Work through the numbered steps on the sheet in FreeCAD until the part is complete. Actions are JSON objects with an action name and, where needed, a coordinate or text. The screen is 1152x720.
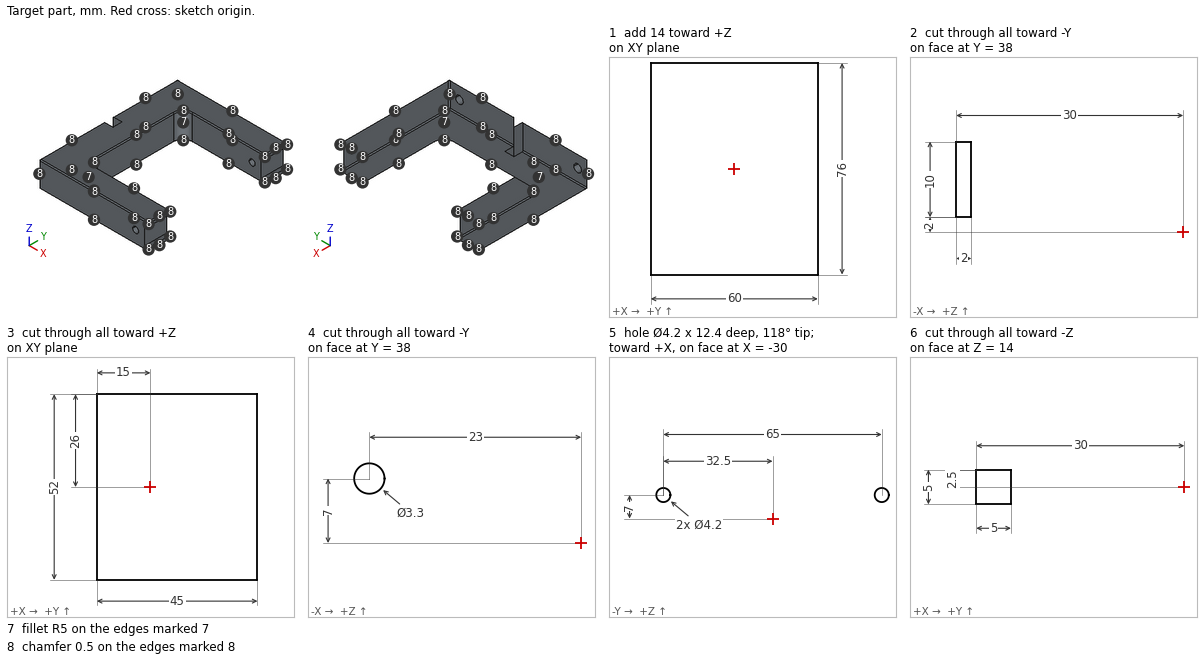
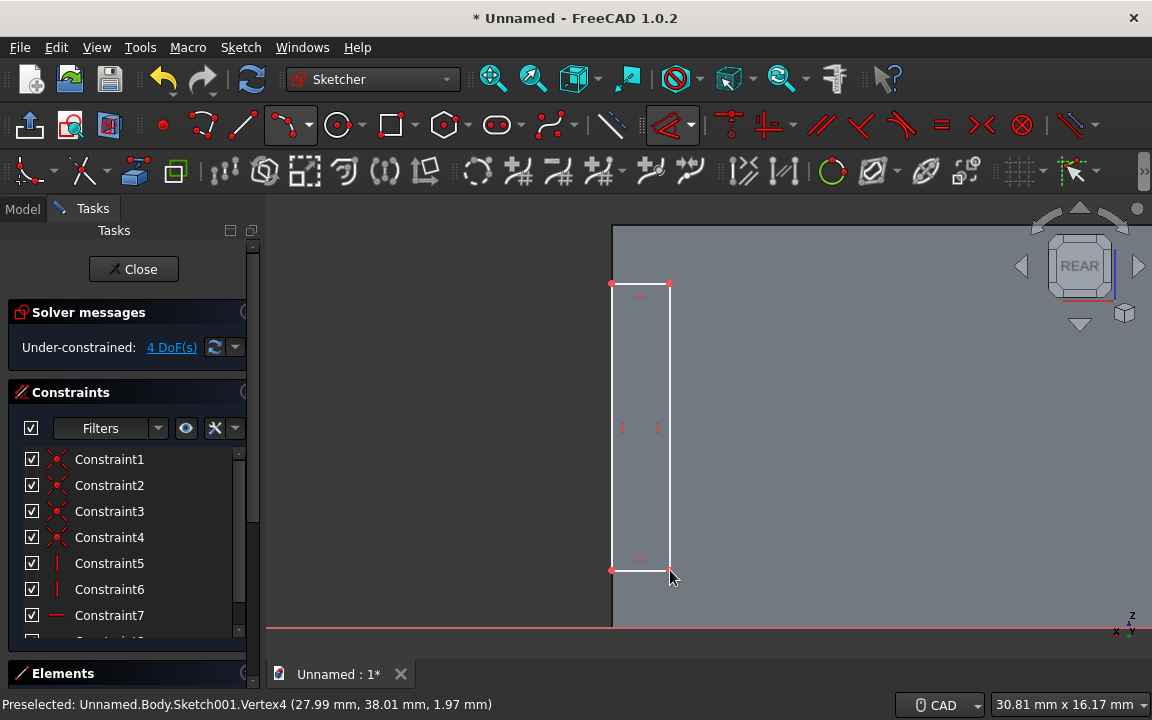
{"action": "left_click", "coordinate": [629, 571]}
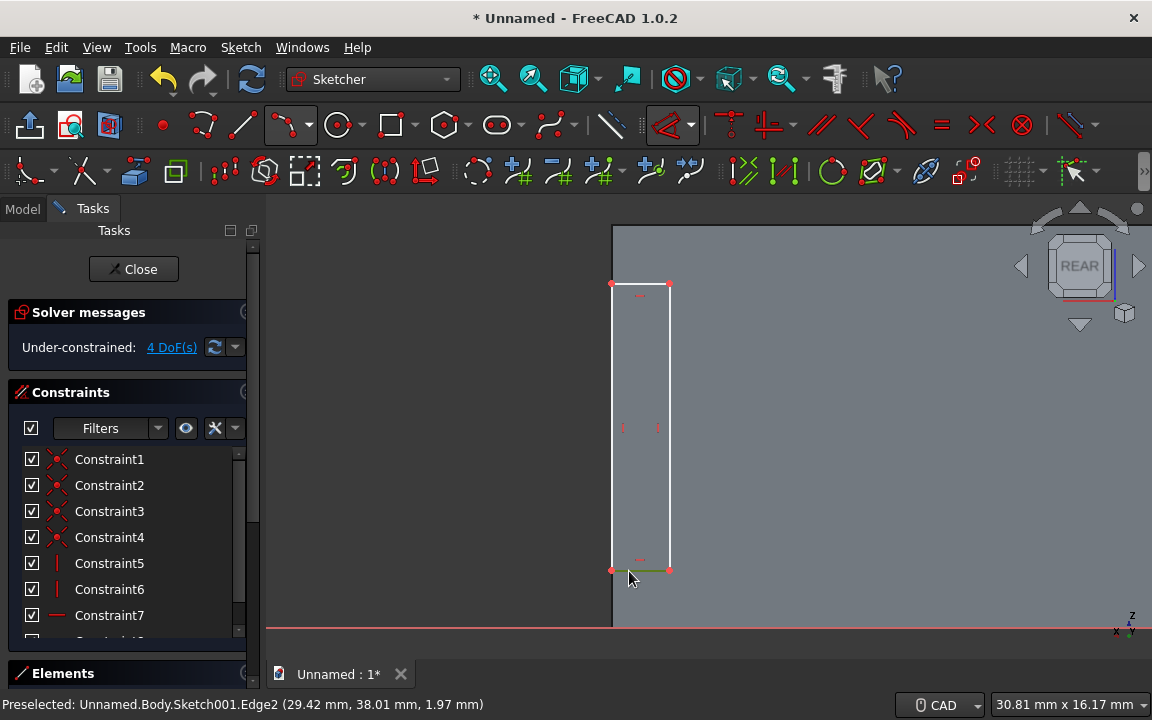
{"action": "key", "text": "l"}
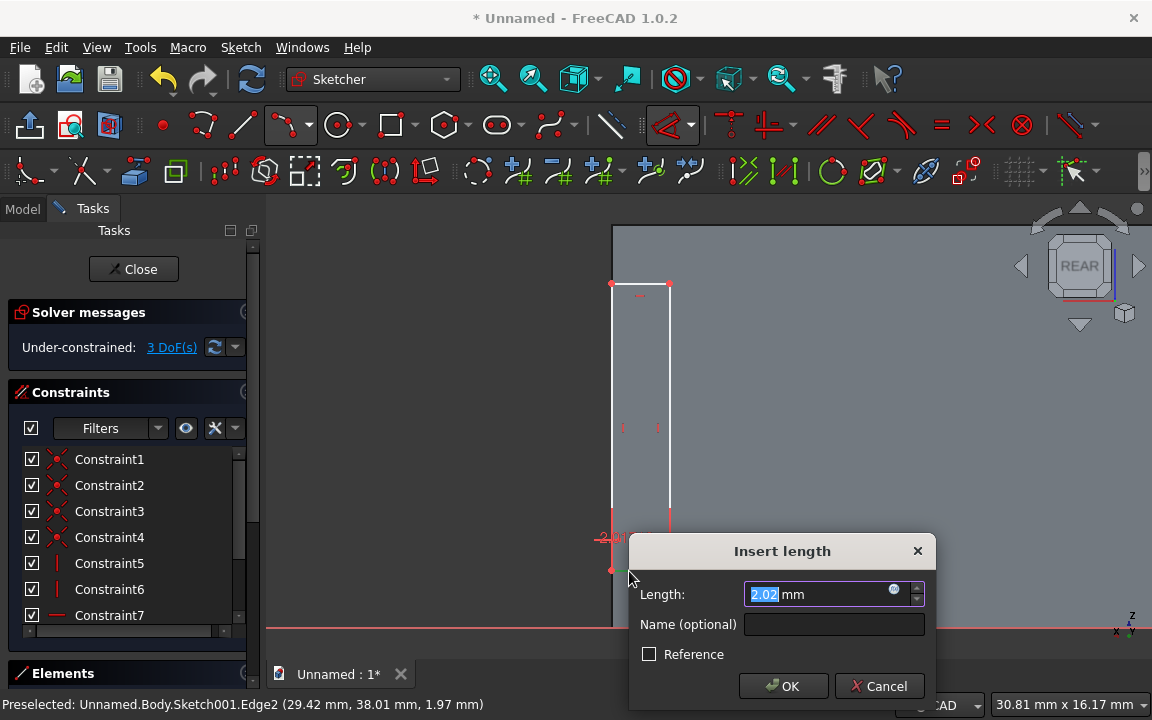
{"action": "type", "text": "2"}
{"action": "key", "text": "Return"}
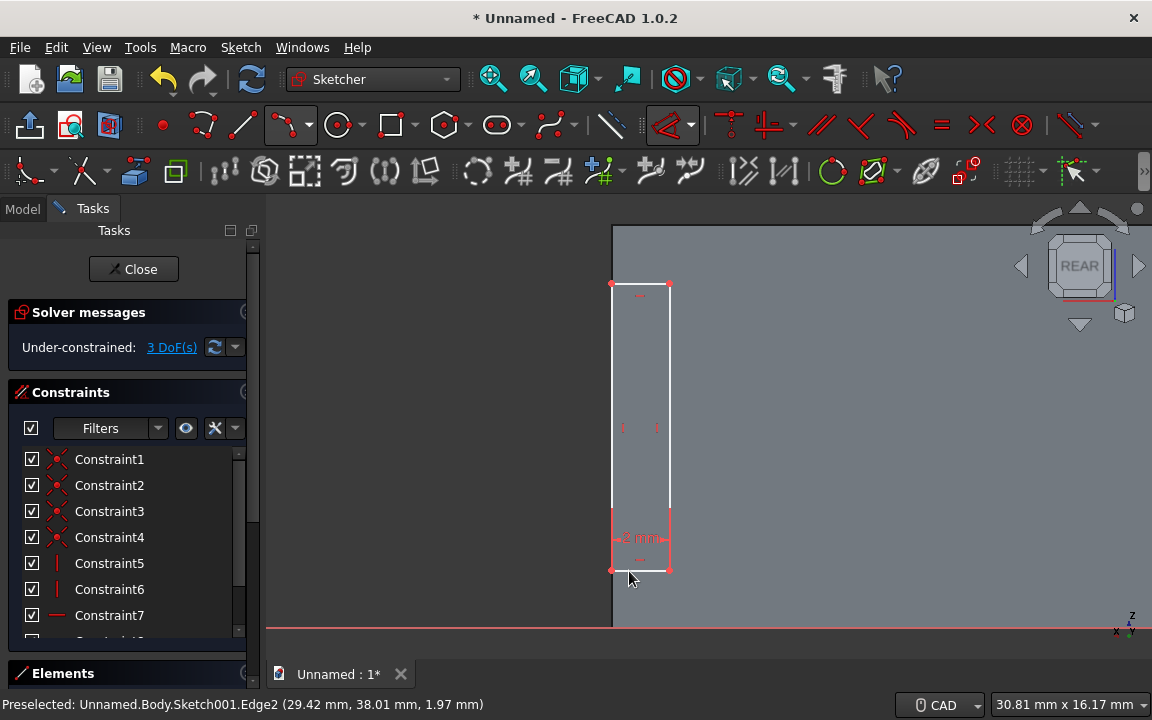
{"action": "left_click", "coordinate": [612, 370]}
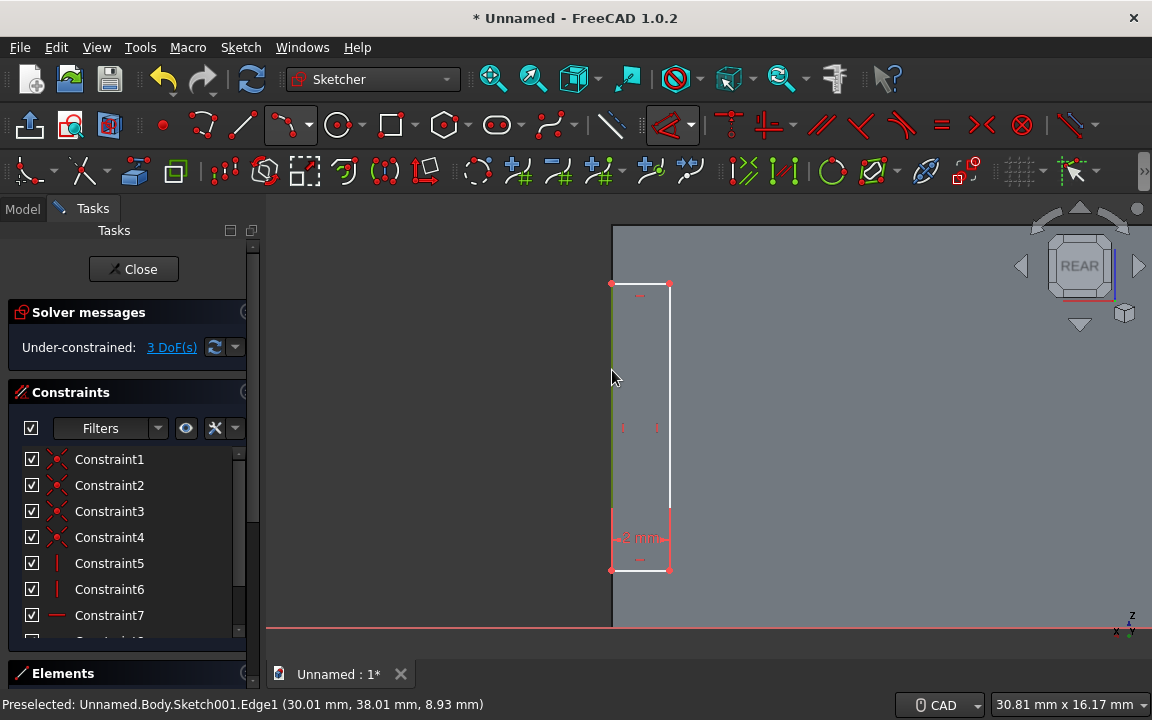
{"action": "key", "text": "i"}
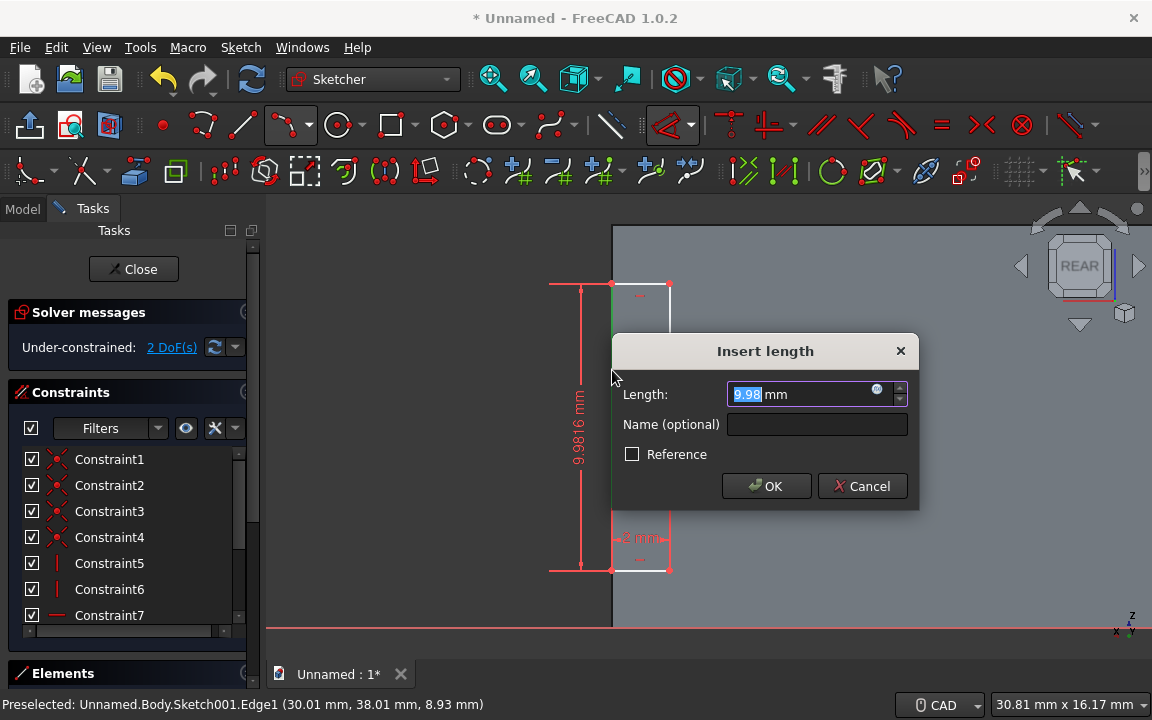
{"action": "type", "text": "10"}
{"action": "key", "text": "Return"}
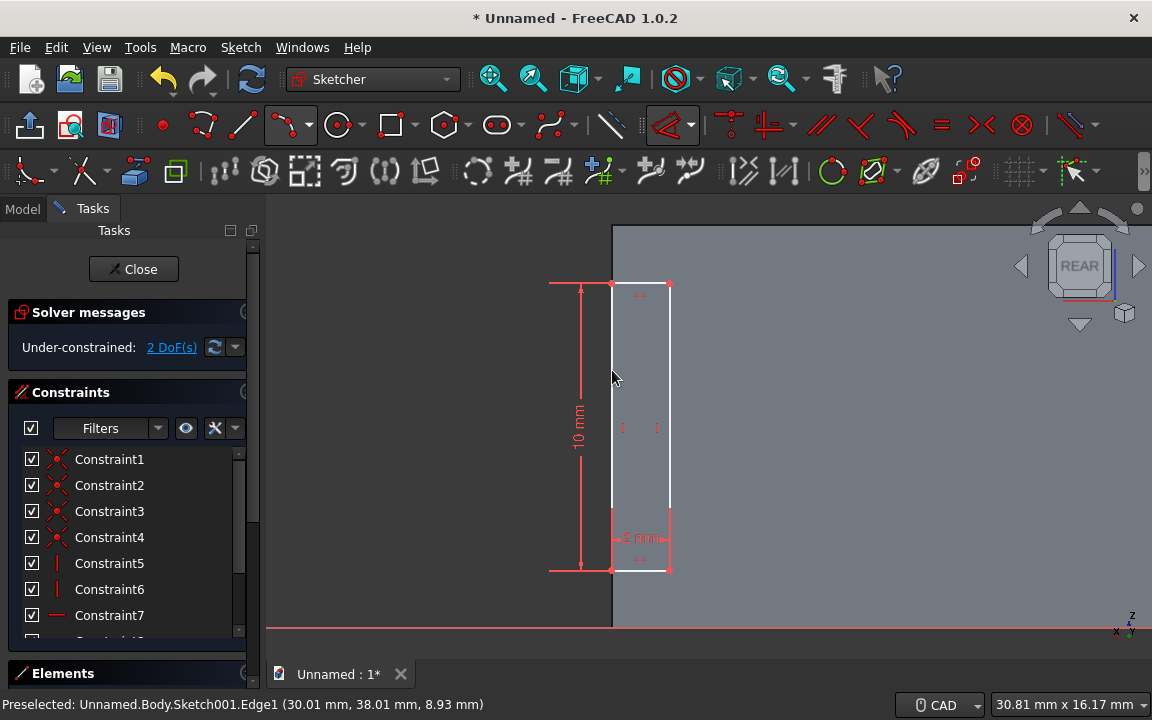
{"action": "left_click", "coordinate": [612, 571]}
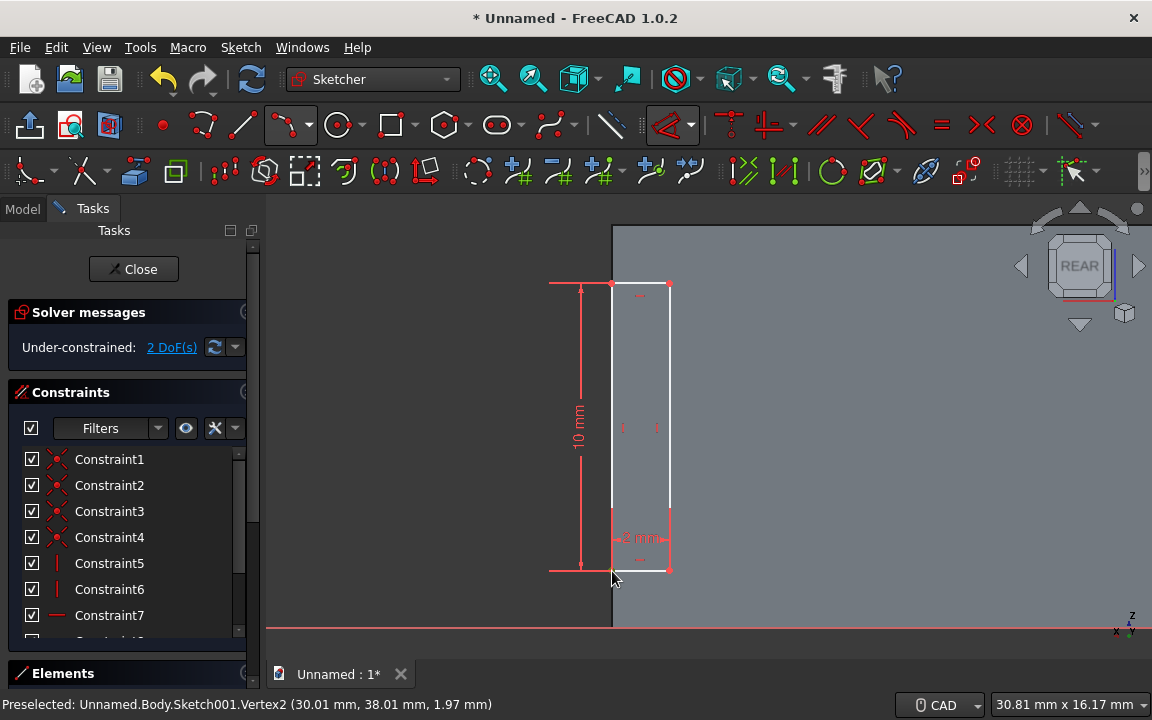
{"action": "key", "text": "i"}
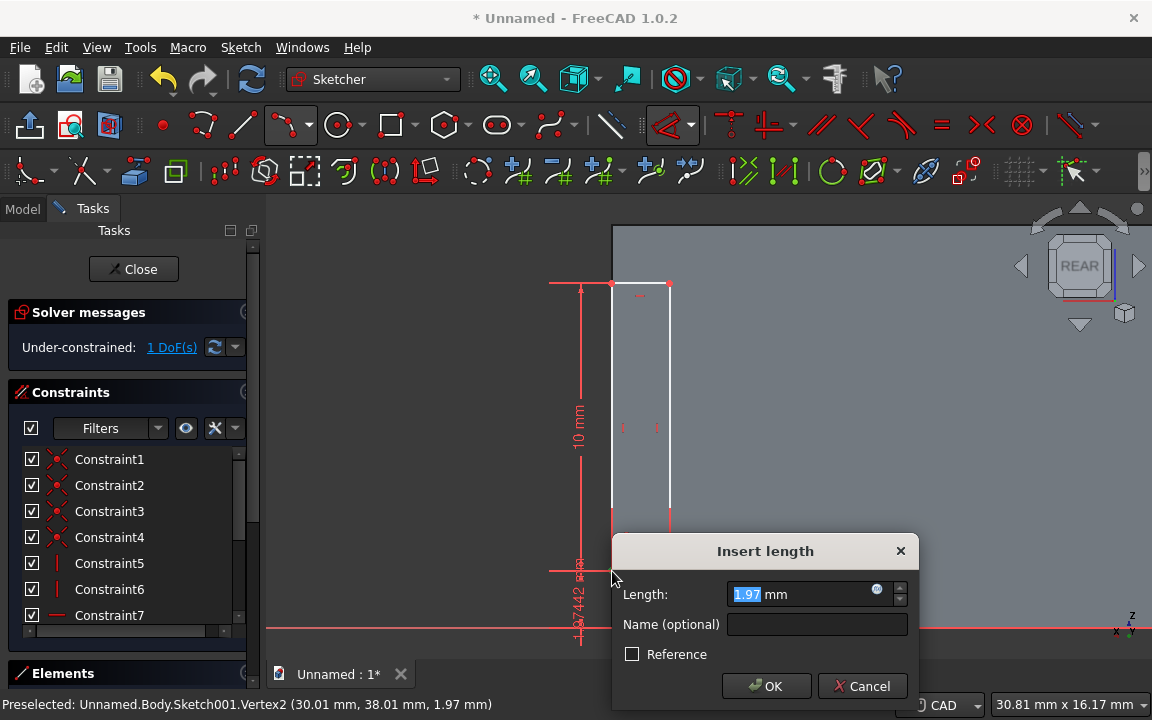
{"action": "type", "text": "2"}
{"action": "key", "text": "Return"}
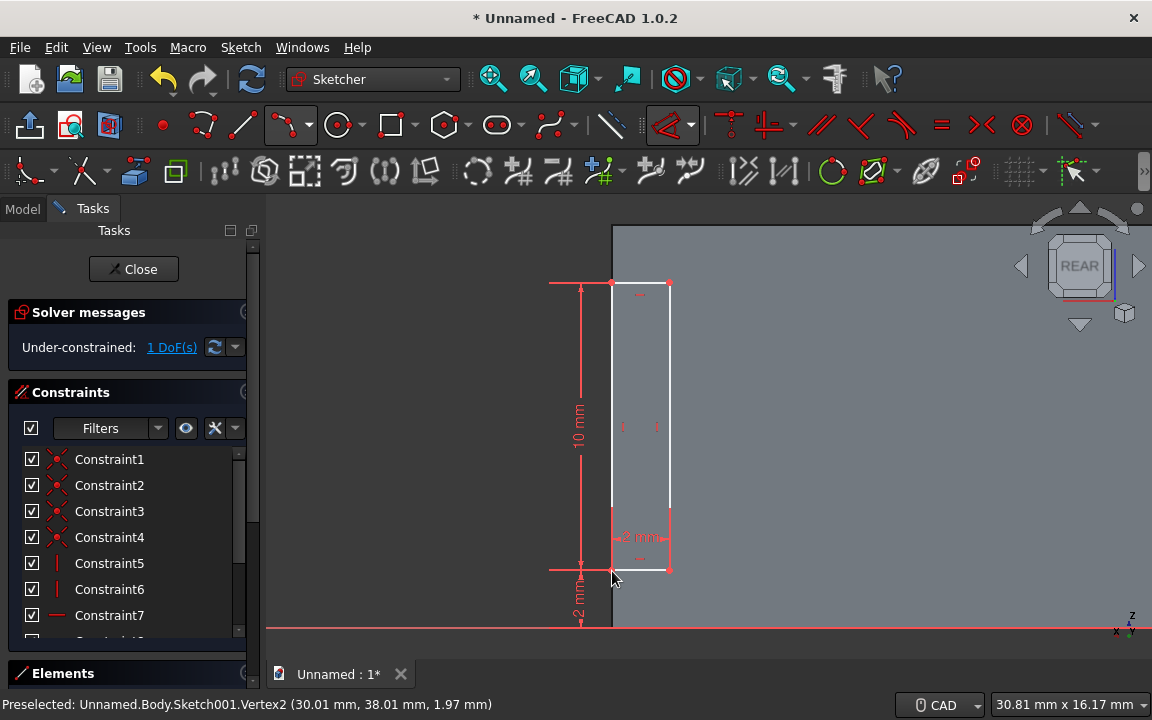
{"action": "left_click", "coordinate": [612, 283]}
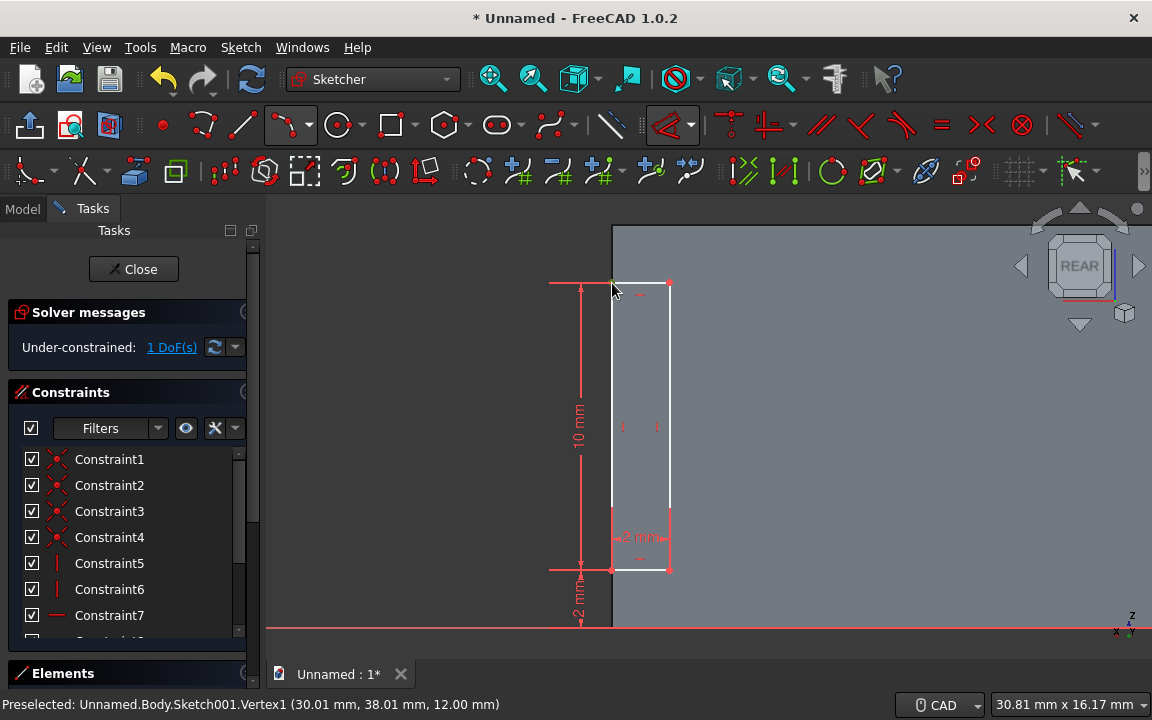
{"action": "key", "text": "l"}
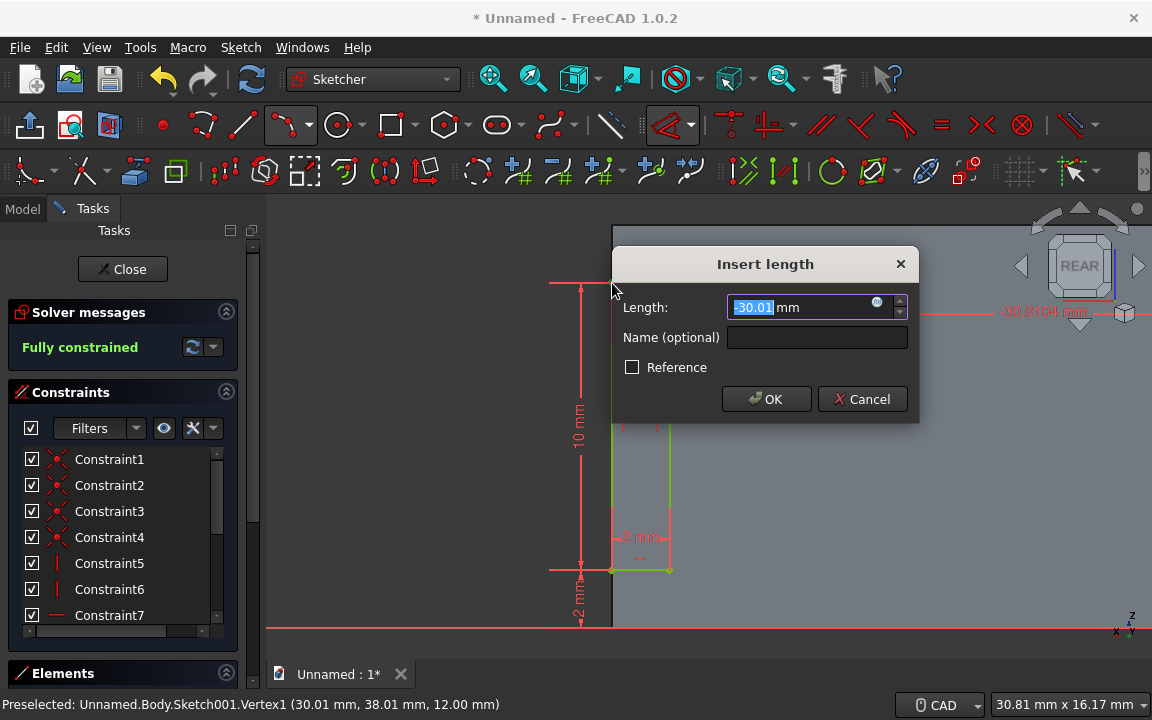
{"action": "type", "text": "-30"}
{"action": "key", "text": "Return"}